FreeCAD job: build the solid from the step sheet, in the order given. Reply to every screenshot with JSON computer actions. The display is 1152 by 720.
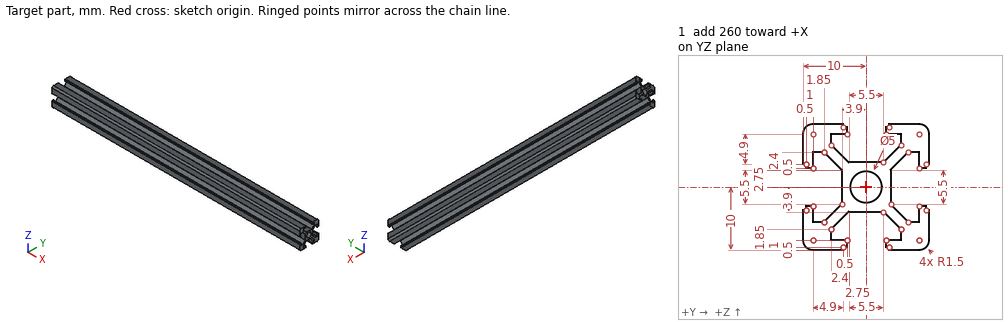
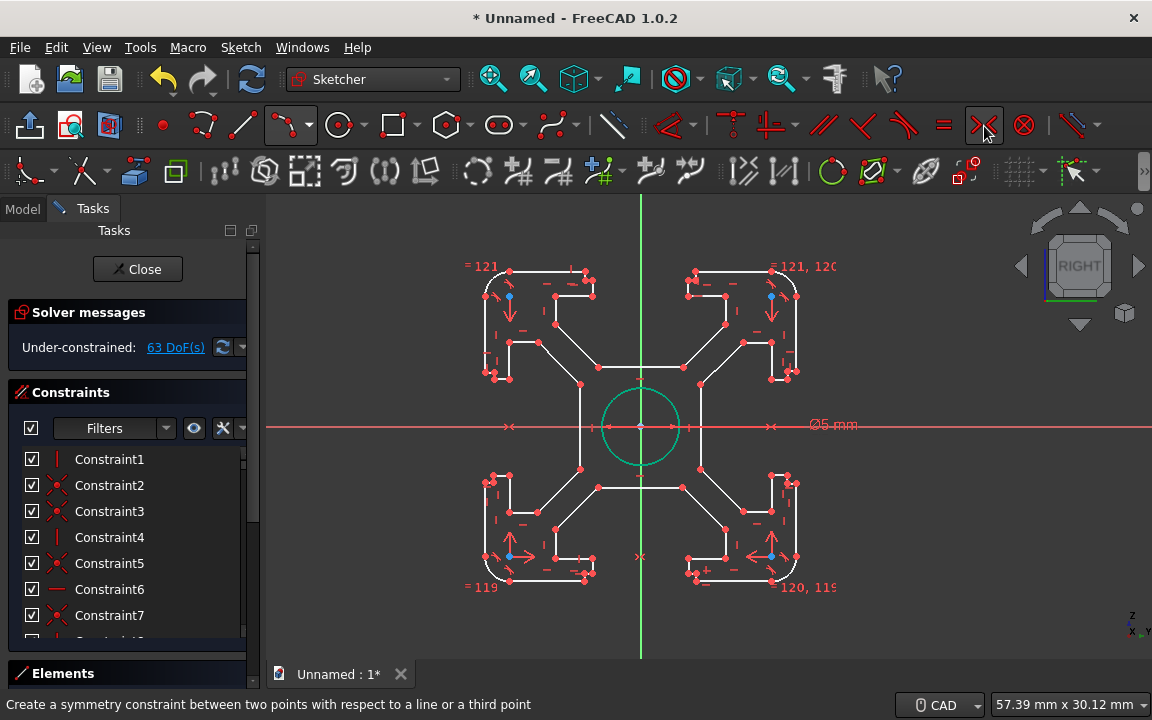
{"action": "left_click", "coordinate": [538, 342]}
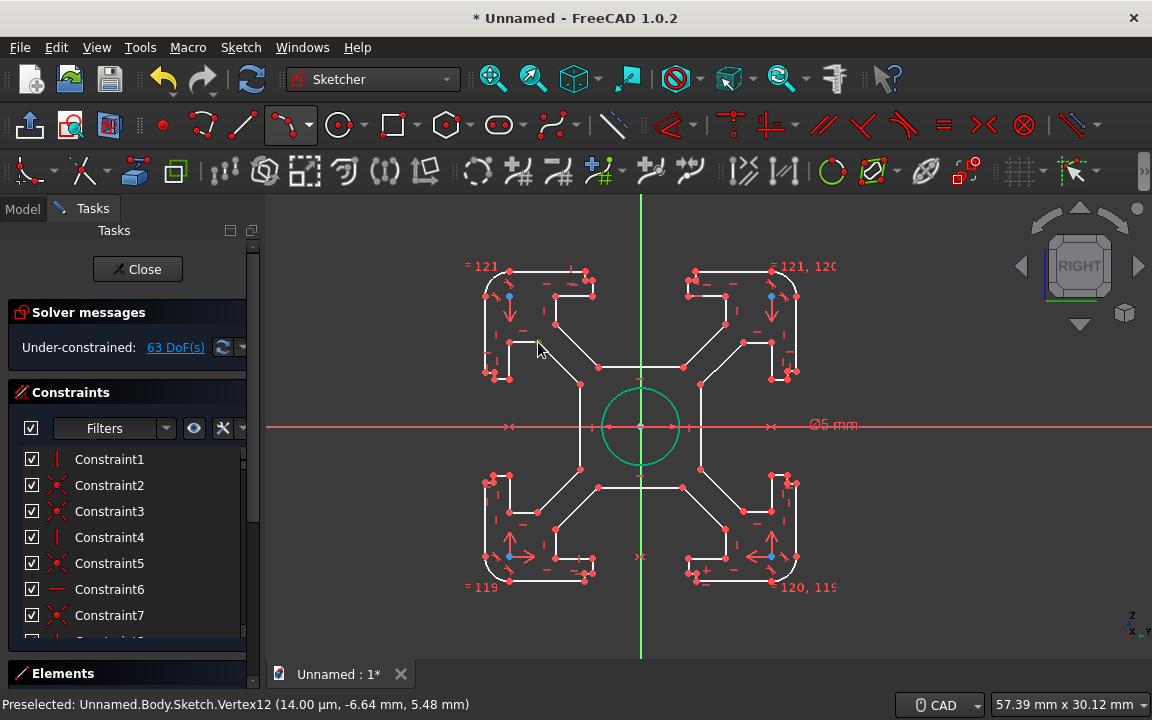
{"action": "left_click", "coordinate": [538, 513]}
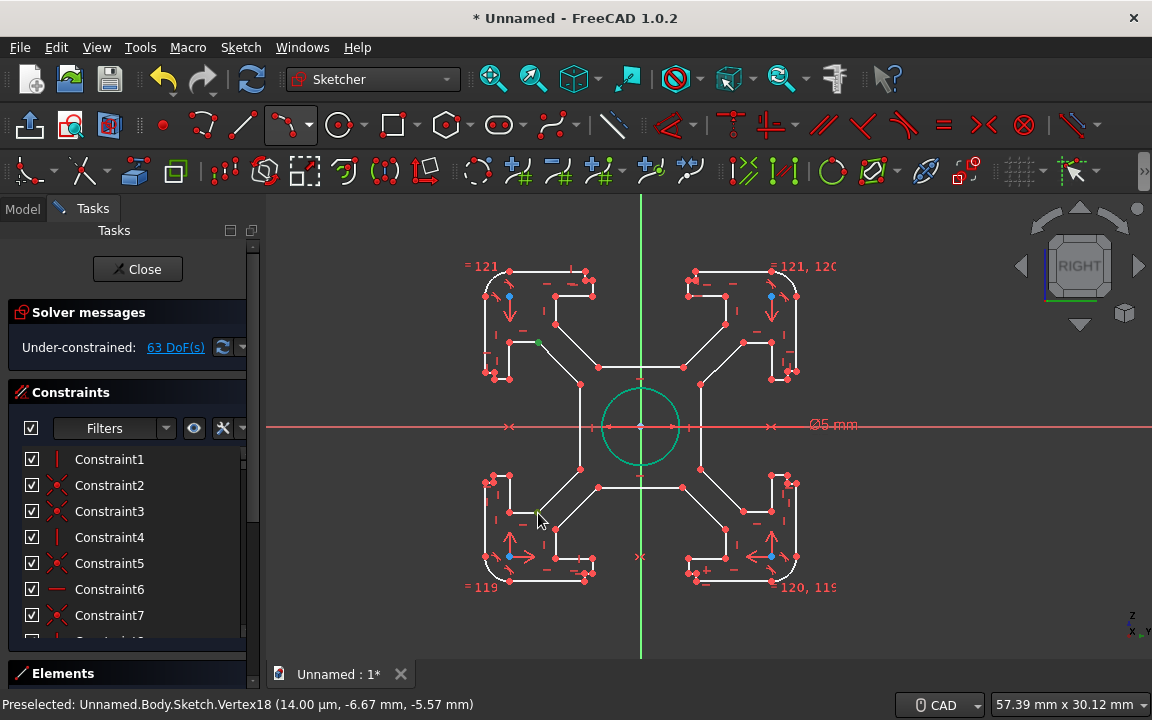
{"action": "left_click", "coordinate": [344, 427]}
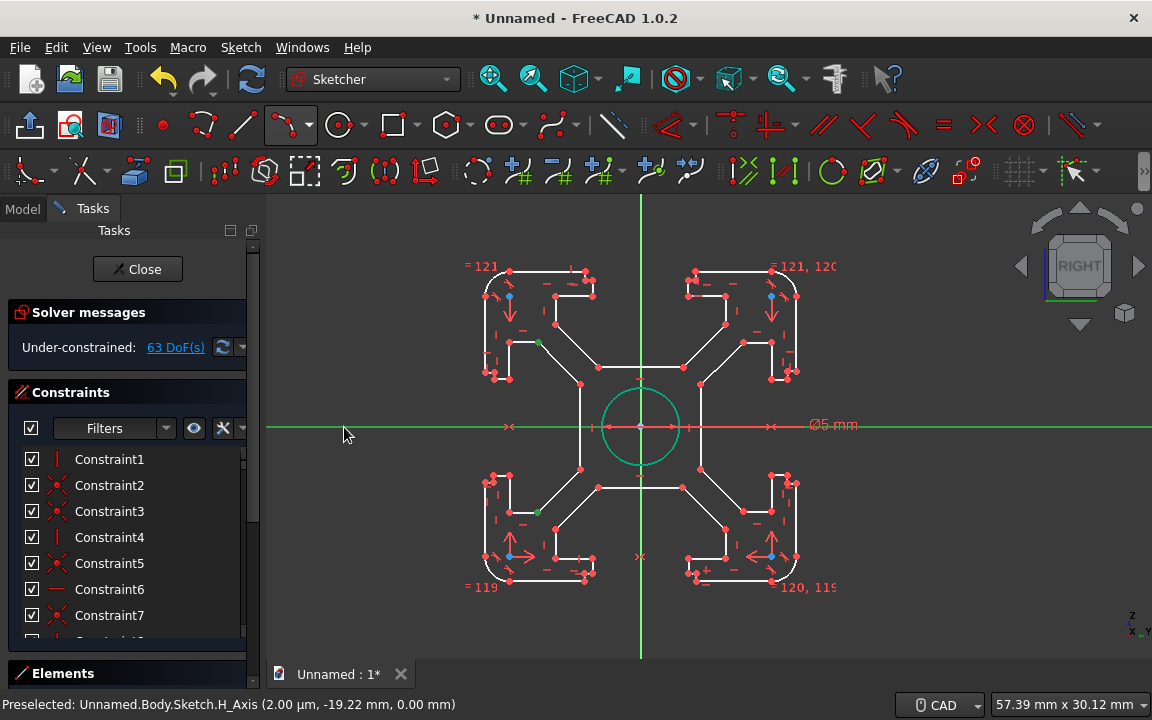
{"action": "key", "text": "s"}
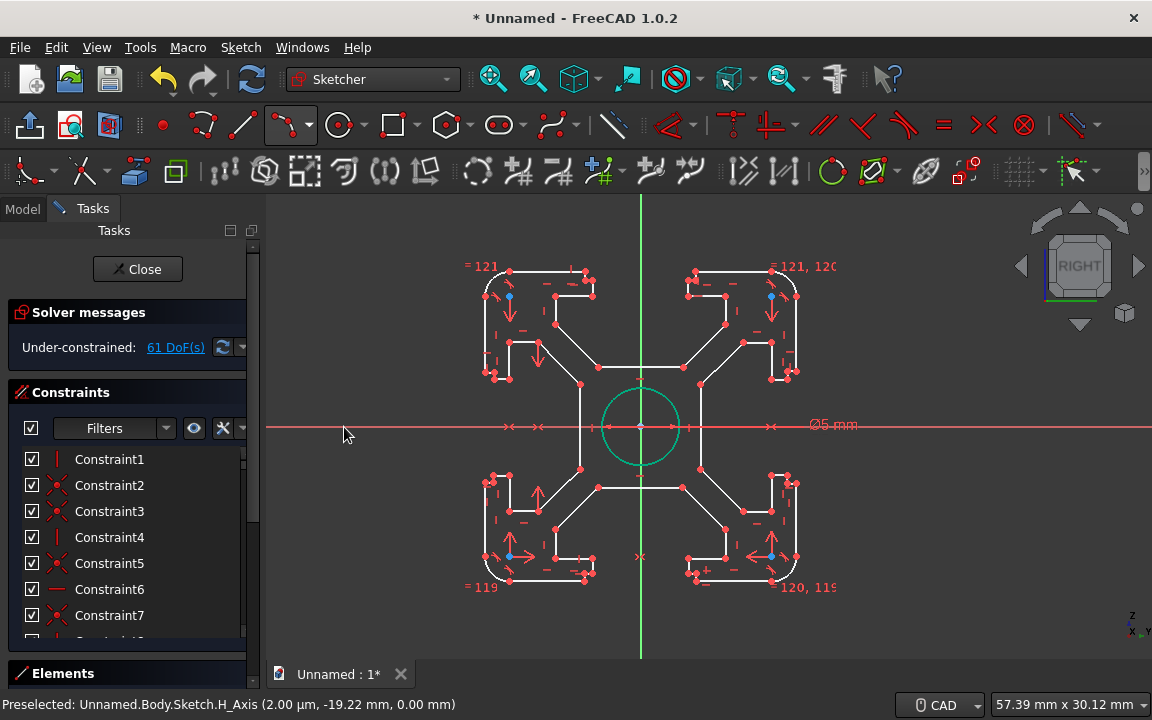
{"action": "left_click", "coordinate": [509, 379]}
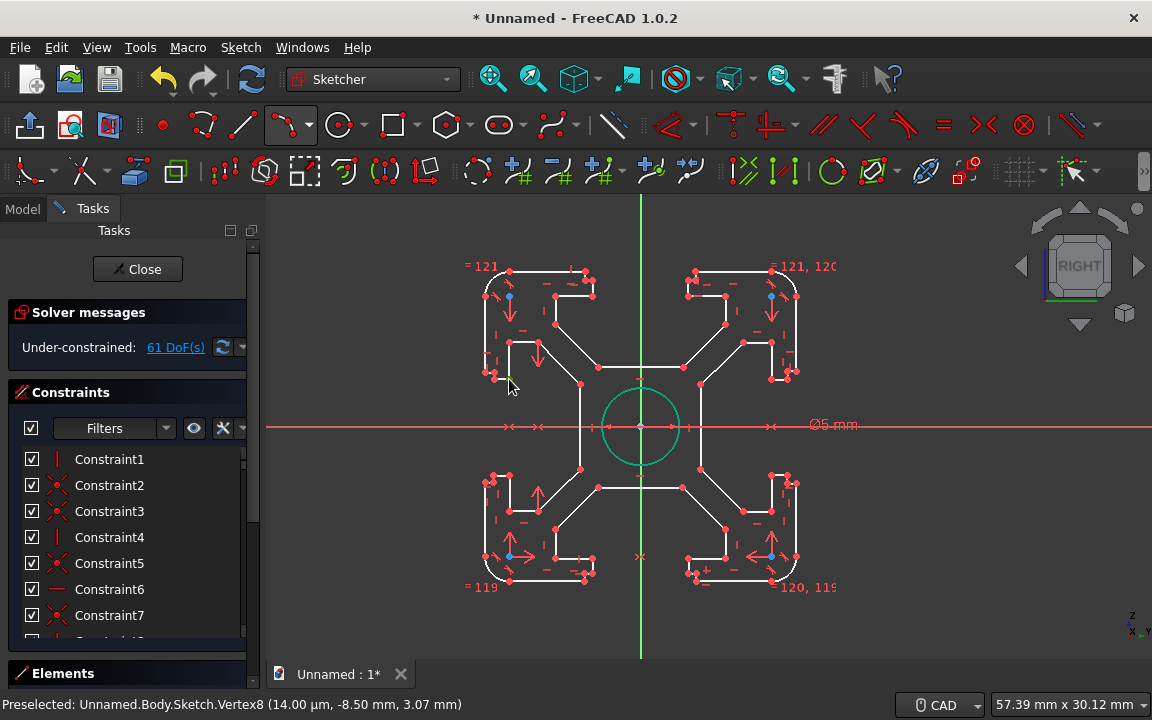
{"action": "left_click", "coordinate": [510, 476]}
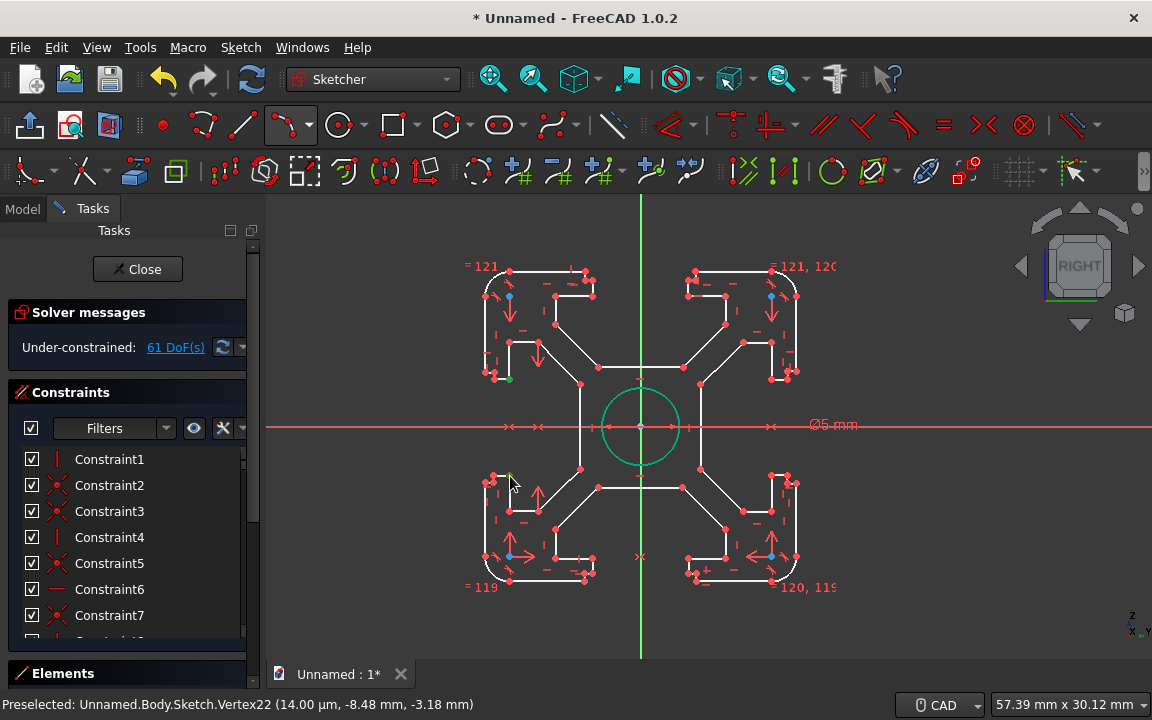
{"action": "left_click", "coordinate": [344, 427]}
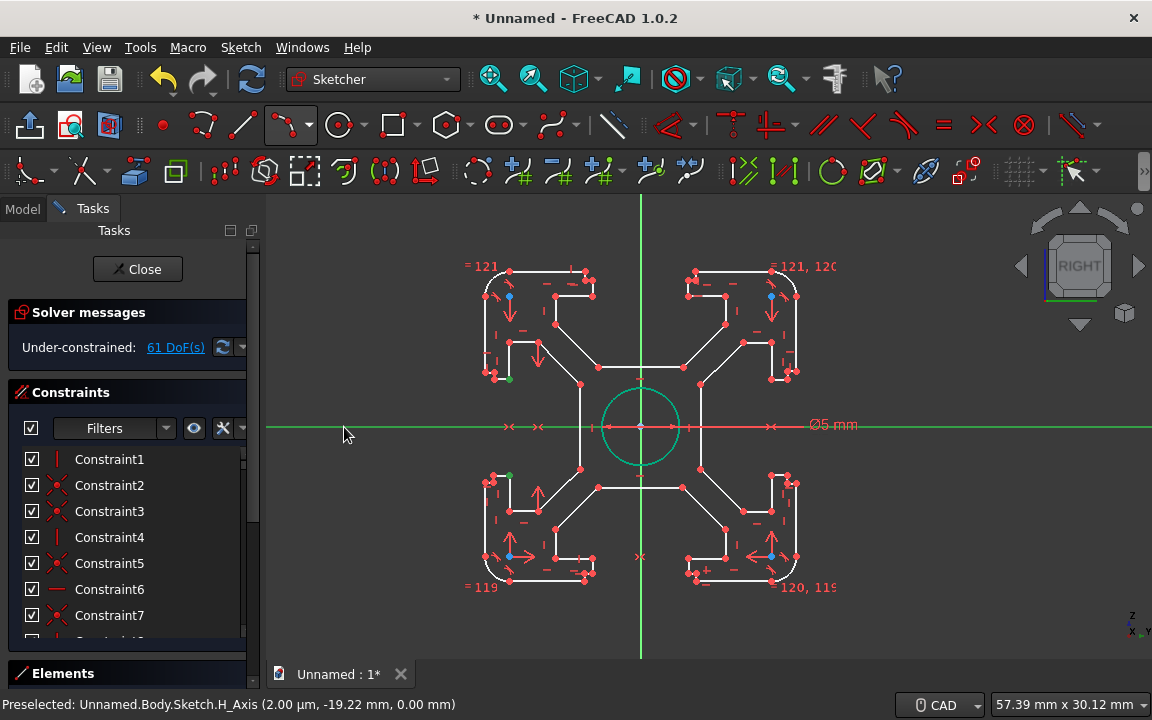
{"action": "left_click", "coordinate": [984, 126]}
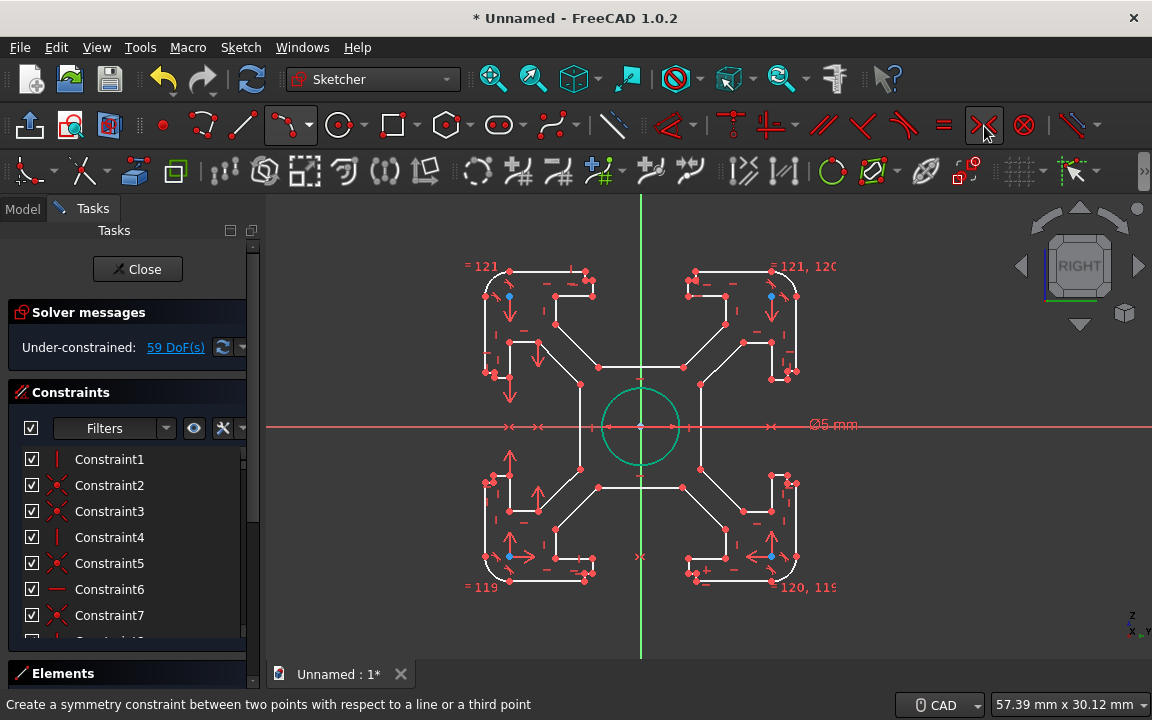
{"action": "scroll", "coordinate": [494, 373], "scroll_direction": "up", "scroll_amount": 5}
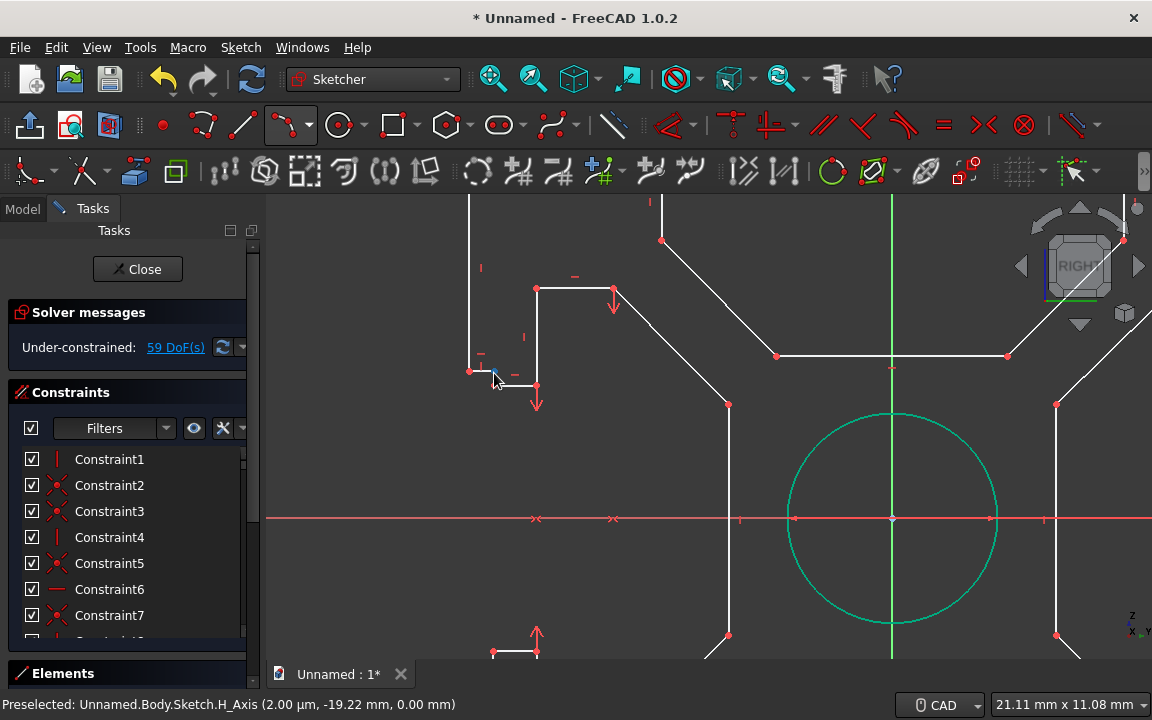
{"action": "left_click", "coordinate": [494, 371]}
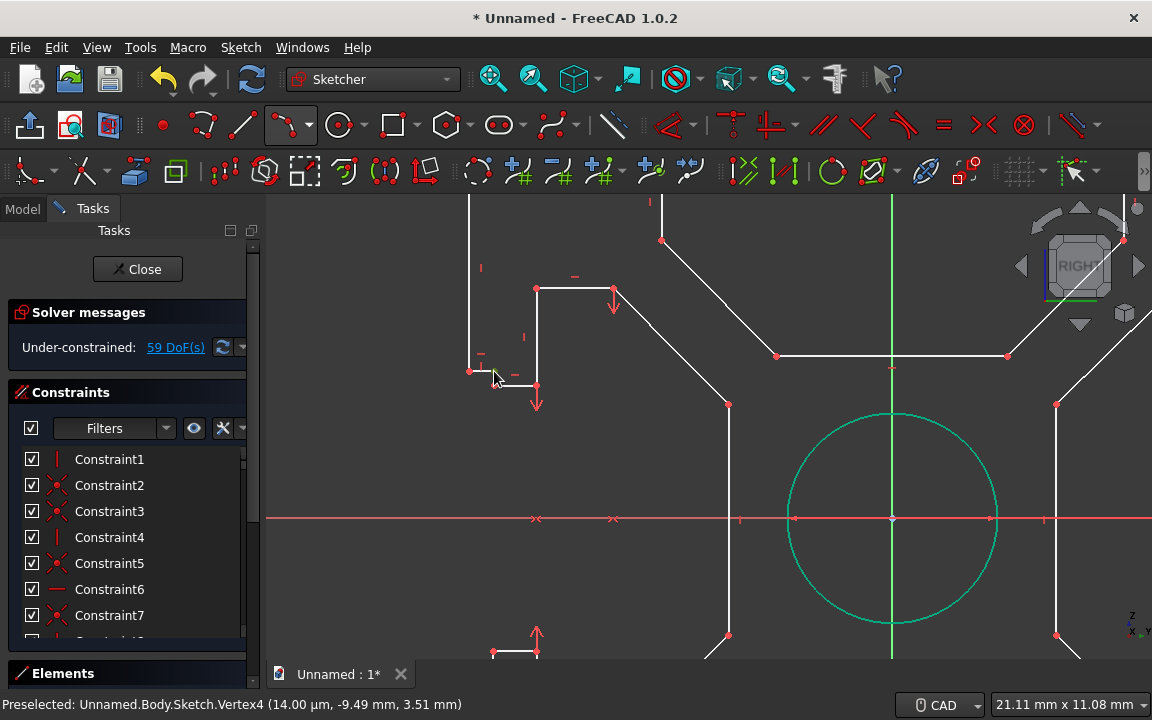
{"action": "scroll", "coordinate": [494, 373], "scroll_direction": "down", "scroll_amount": 5}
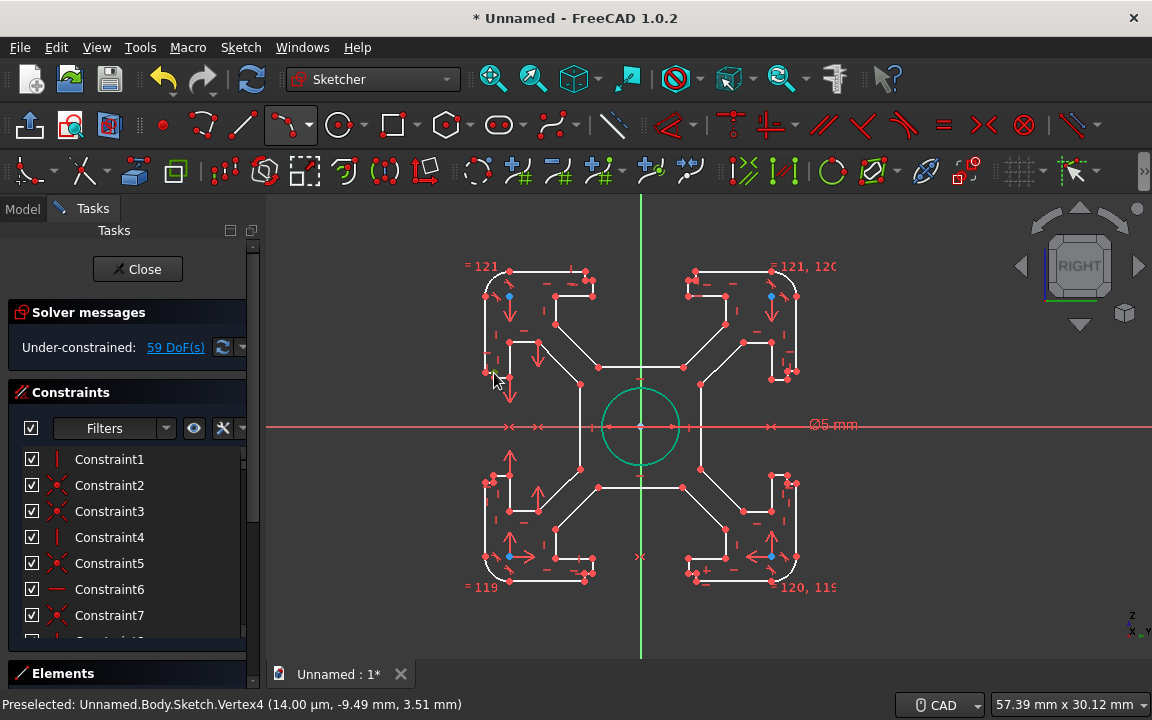
{"action": "scroll", "coordinate": [494, 483], "scroll_direction": "up", "scroll_amount": 3}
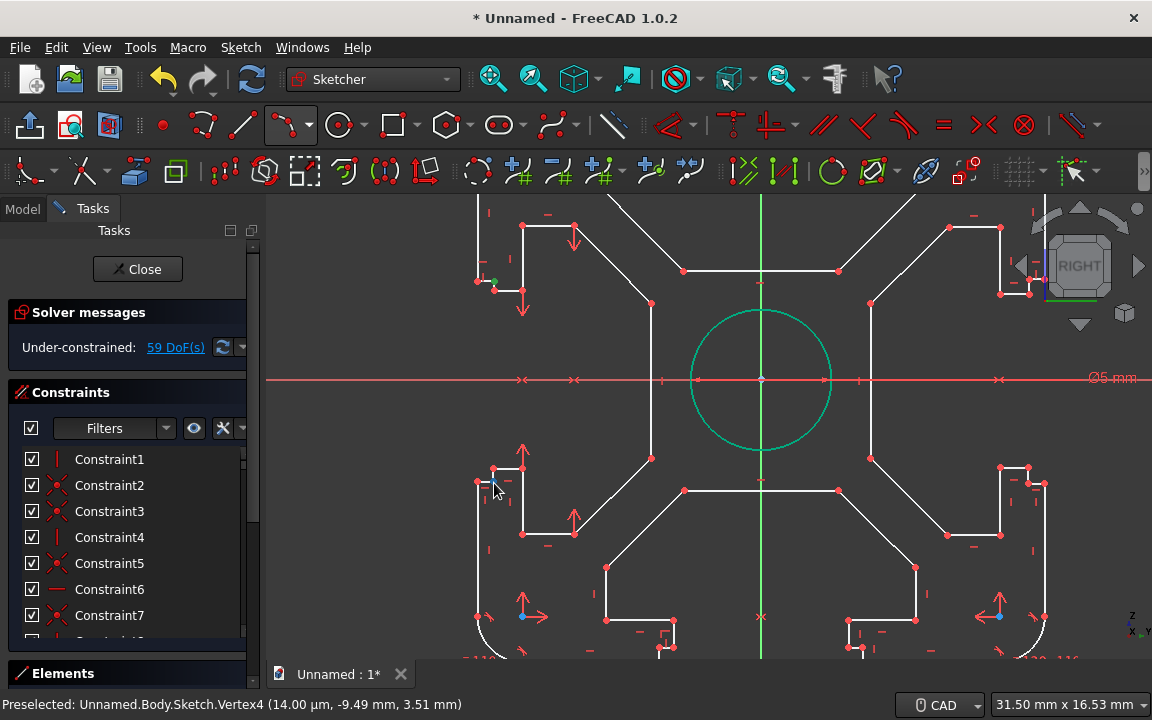
{"action": "left_click", "coordinate": [493, 482]}